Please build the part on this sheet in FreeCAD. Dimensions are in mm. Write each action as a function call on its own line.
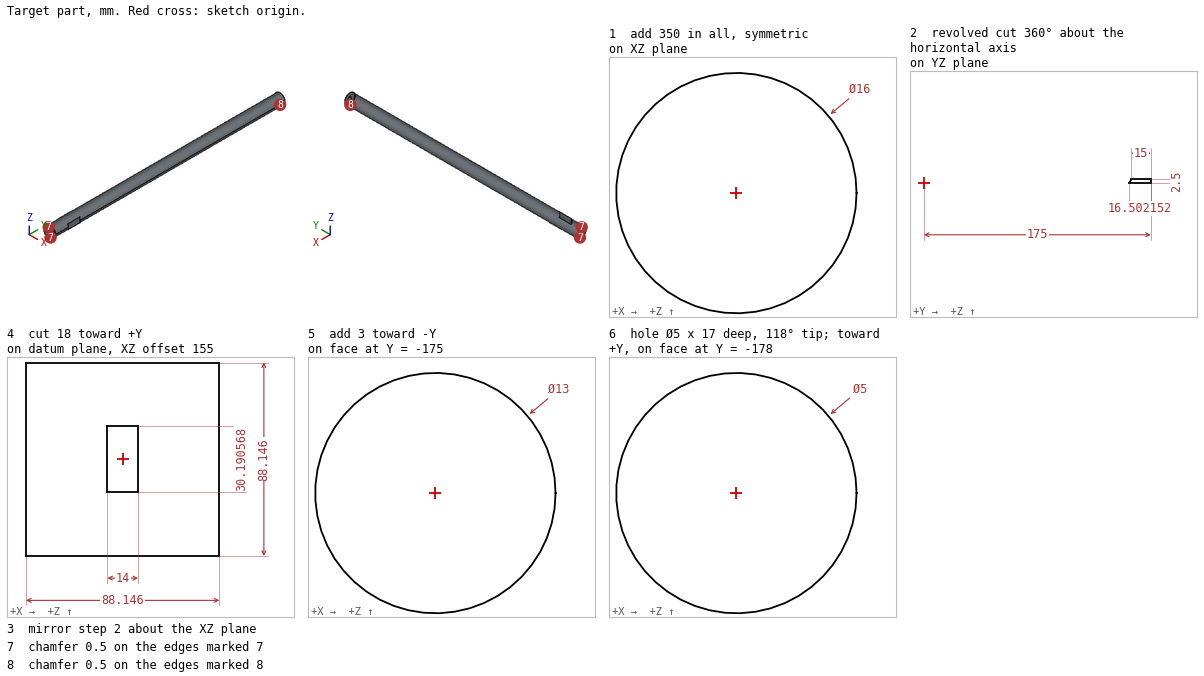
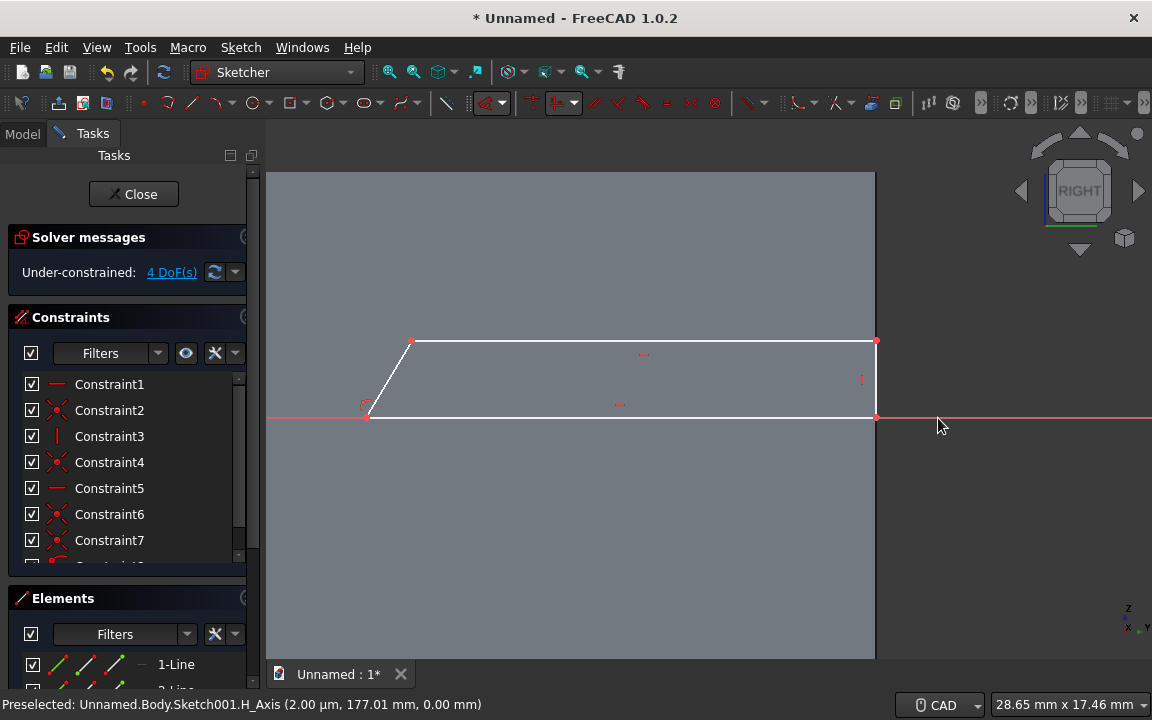
click(486, 104)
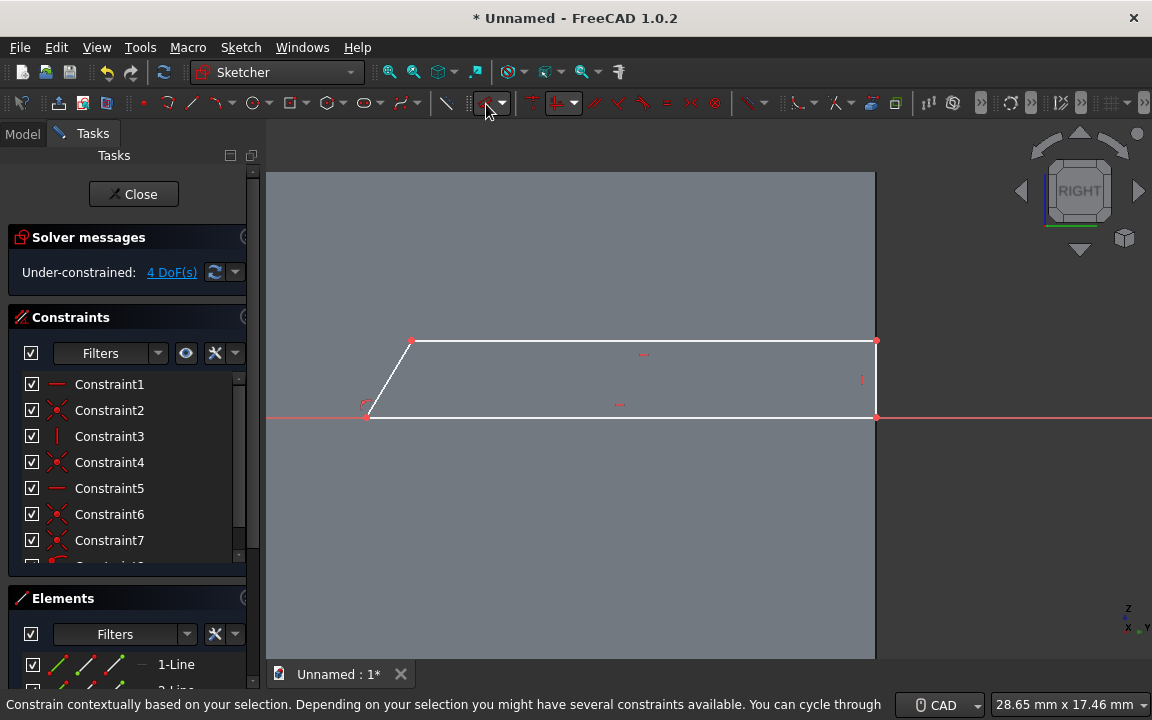
click(737, 341)
click(644, 307)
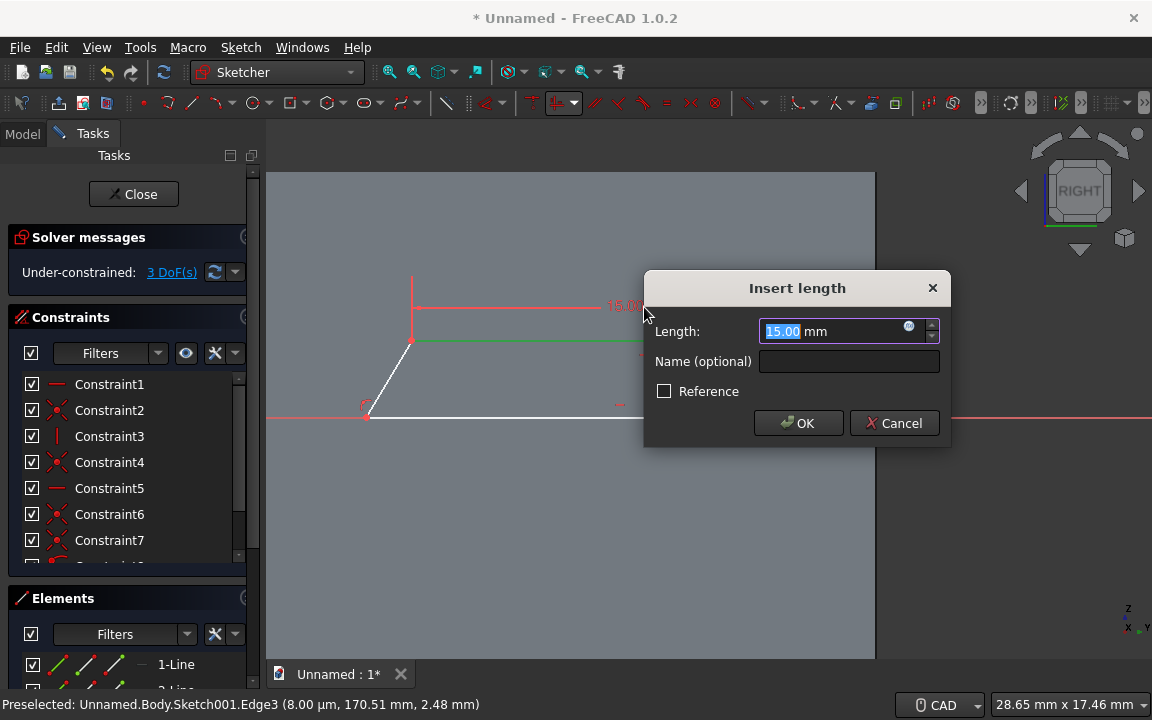
text(15)
key(Return)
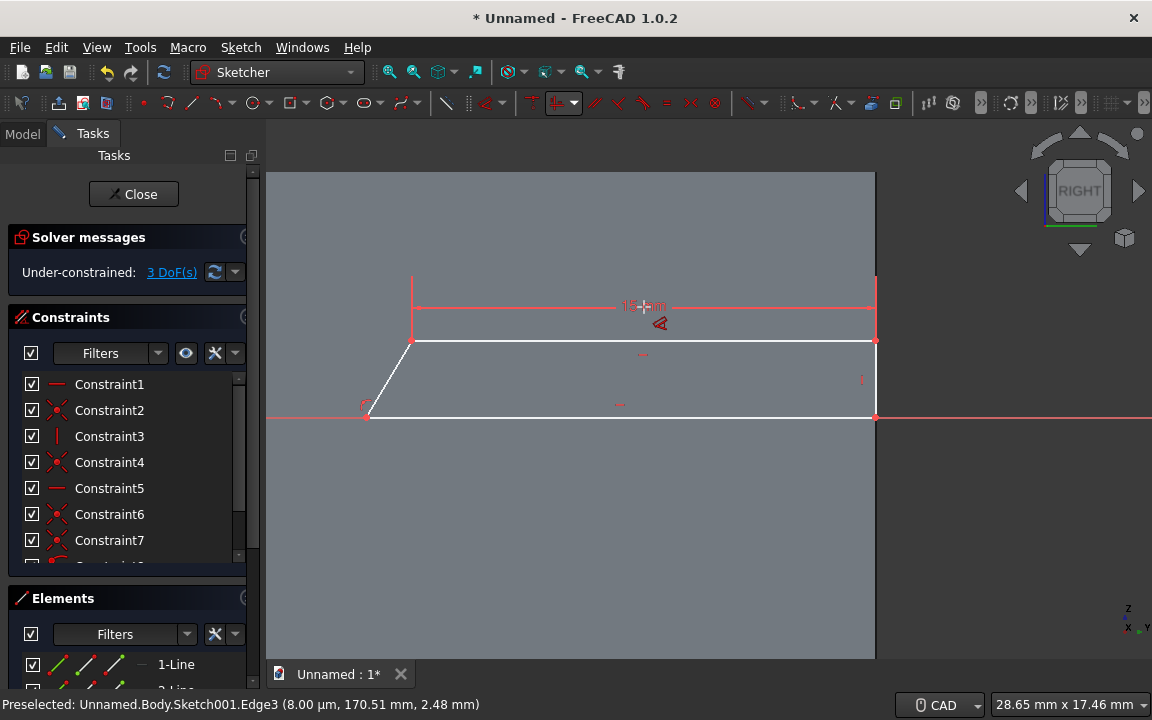
click(876, 395)
click(910, 379)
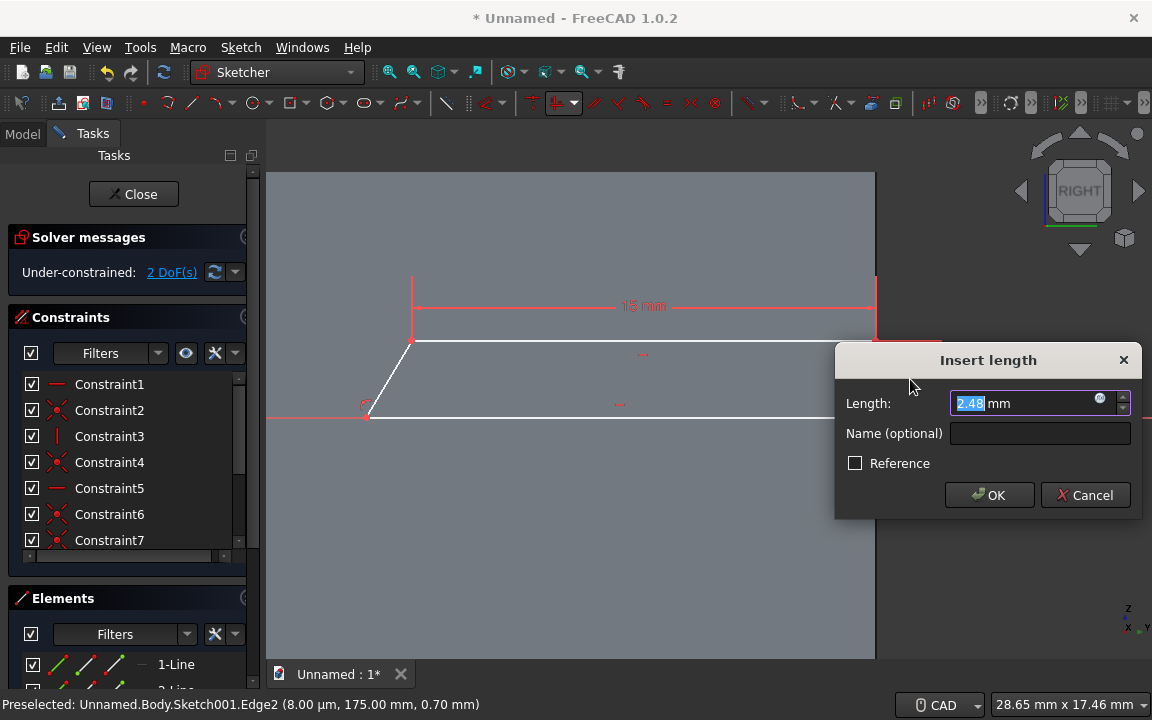
text(2.5)
key(Return)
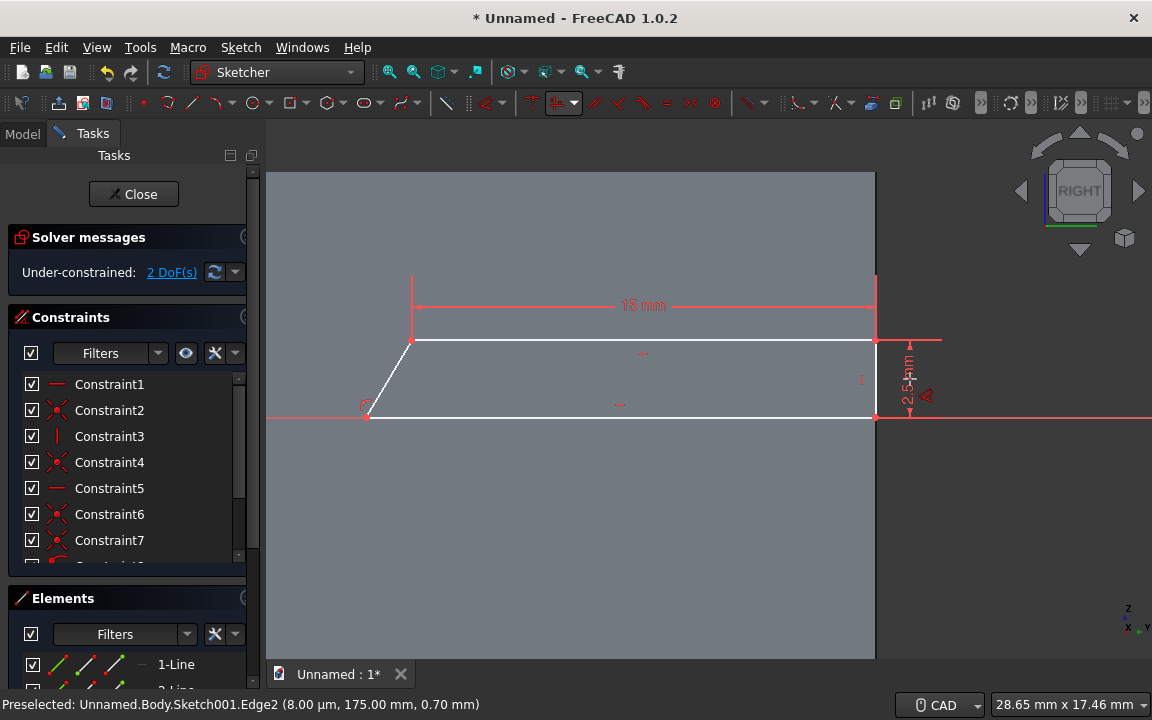
click(876, 418)
click(585, 452)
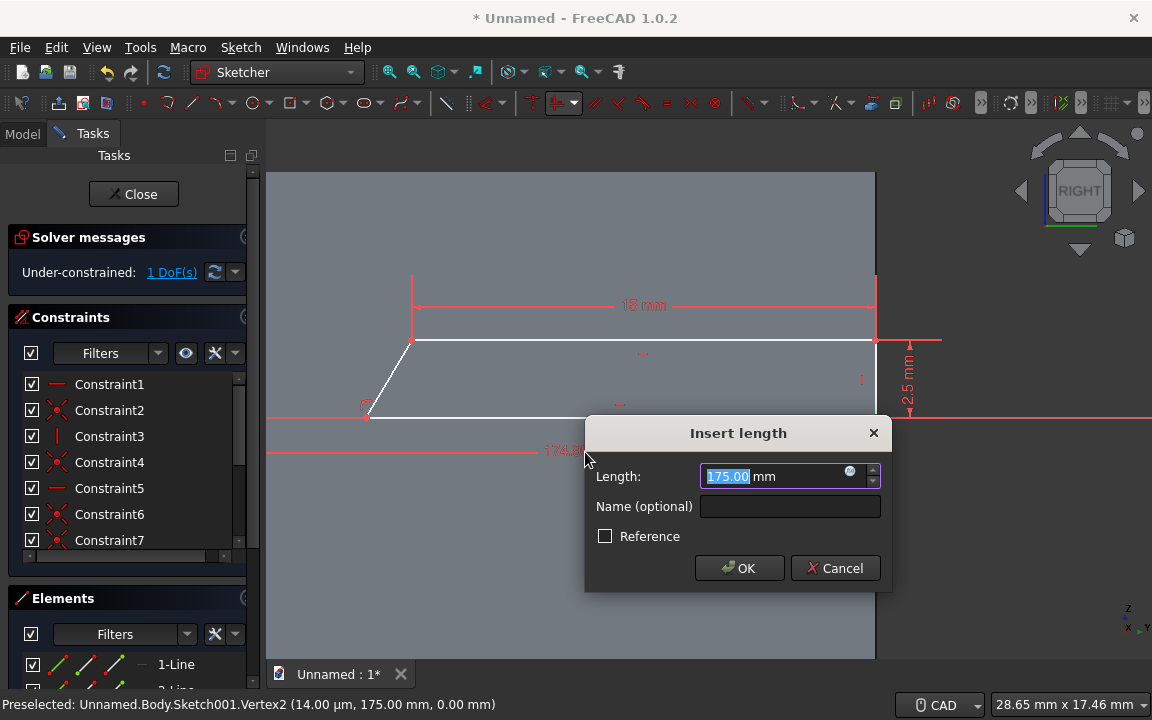
text(175)
key(Return)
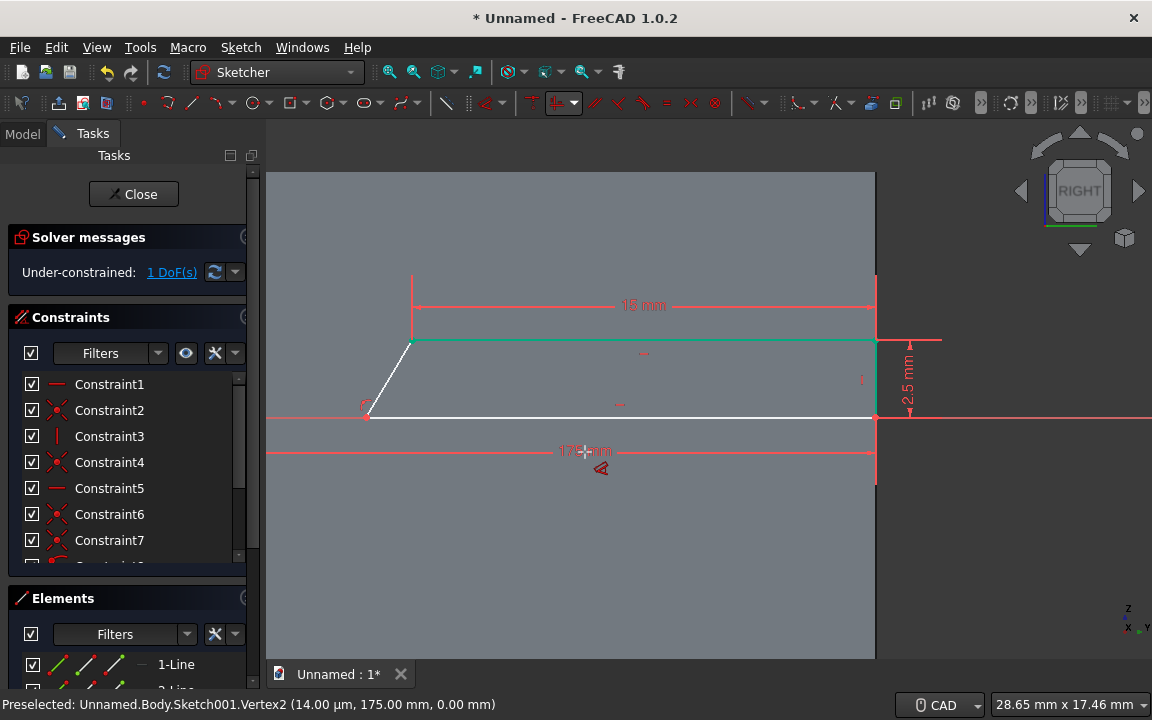
click(519, 418)
click(504, 452)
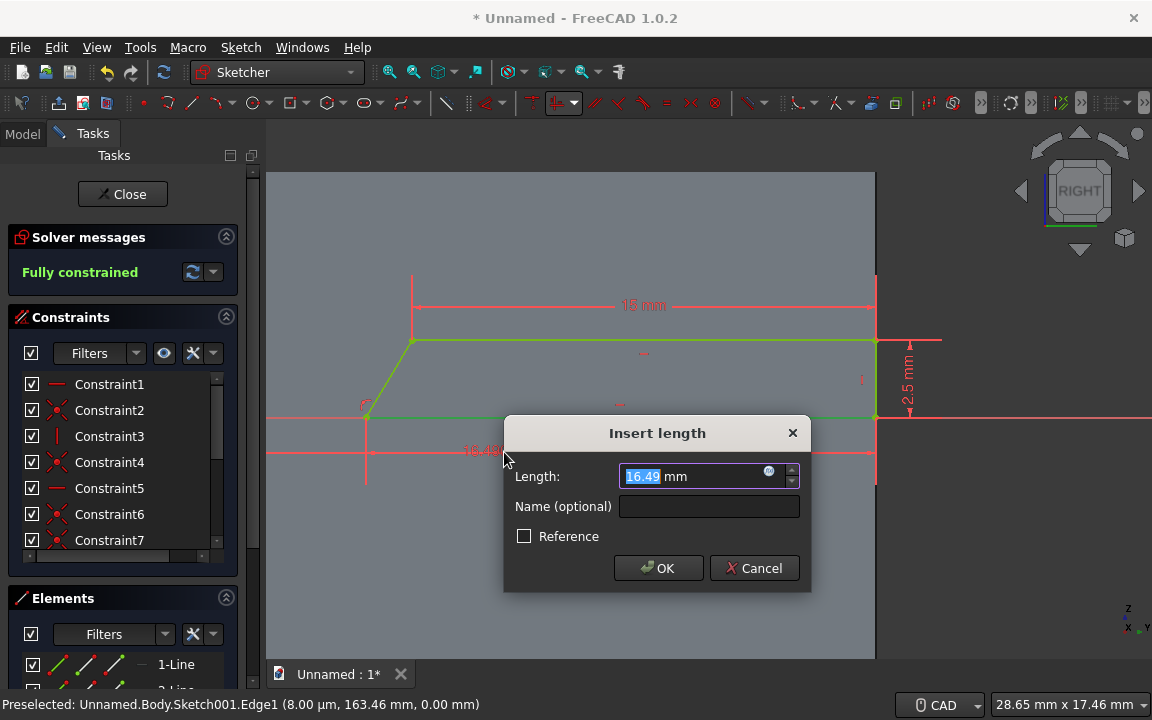
text(16.502152)
key(Return)
key(Escape)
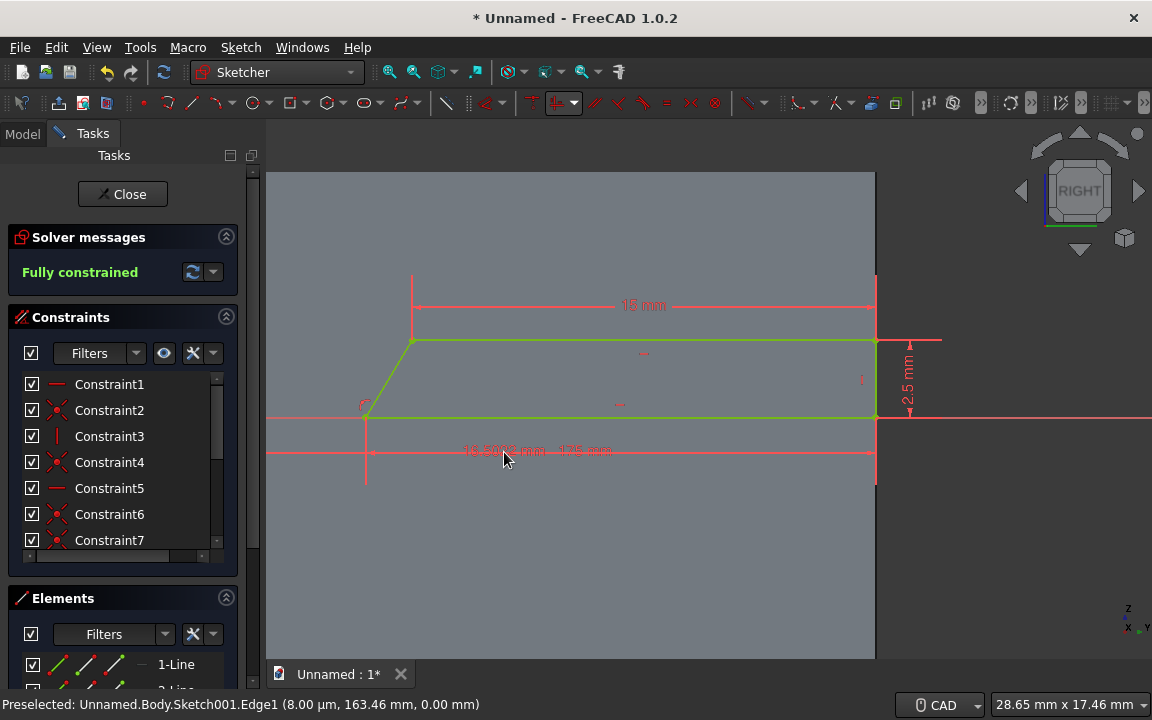
click(123, 194)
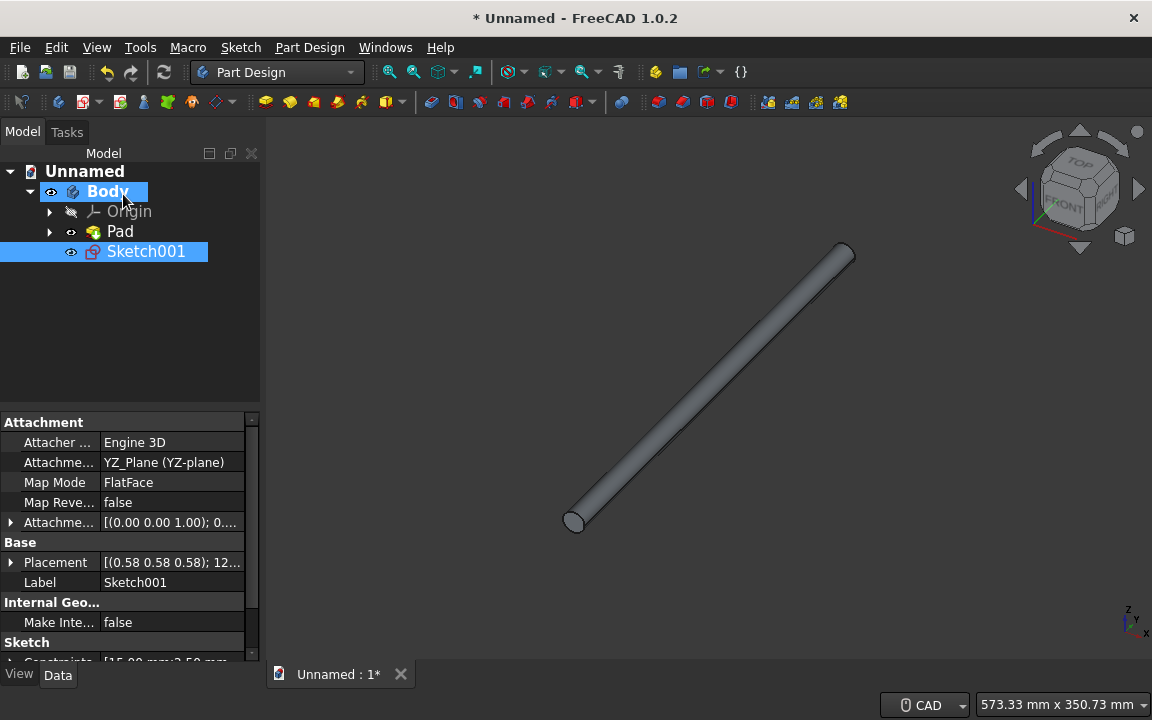
click(480, 102)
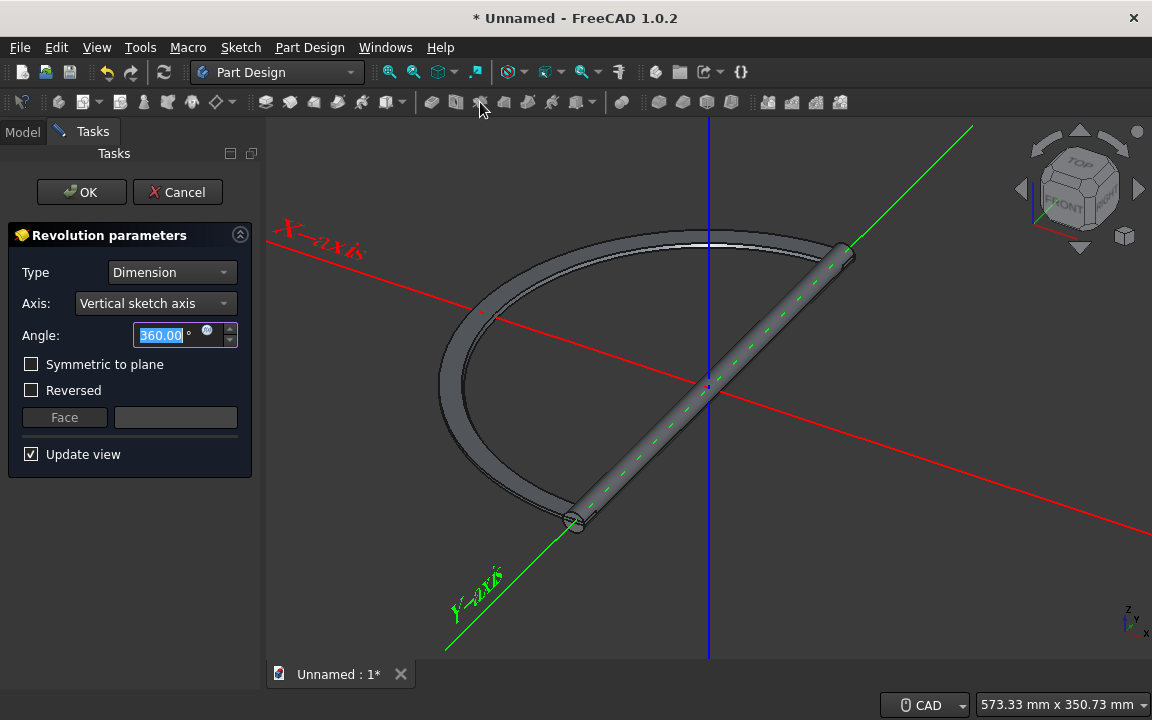
click(156, 304)